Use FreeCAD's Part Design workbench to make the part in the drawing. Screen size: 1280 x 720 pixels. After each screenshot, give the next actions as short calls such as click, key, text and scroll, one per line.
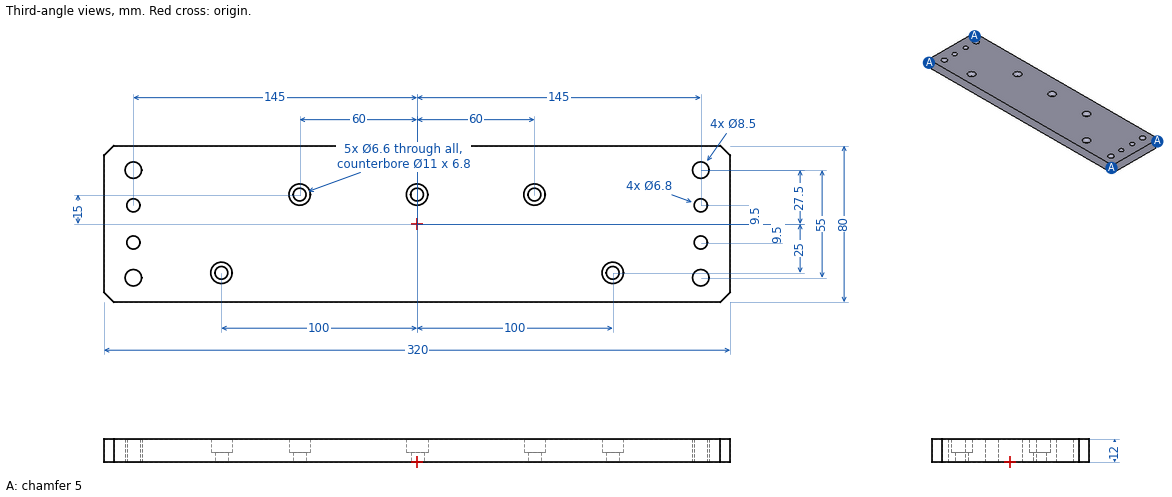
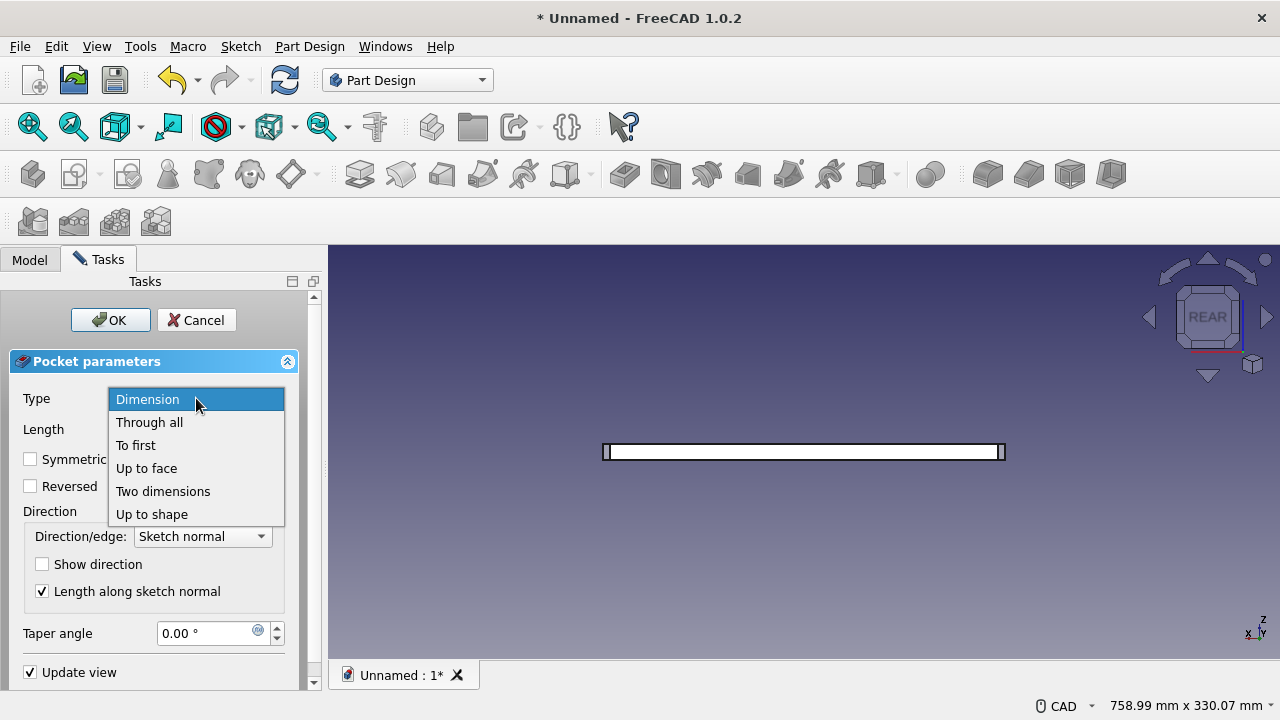
click(194, 422)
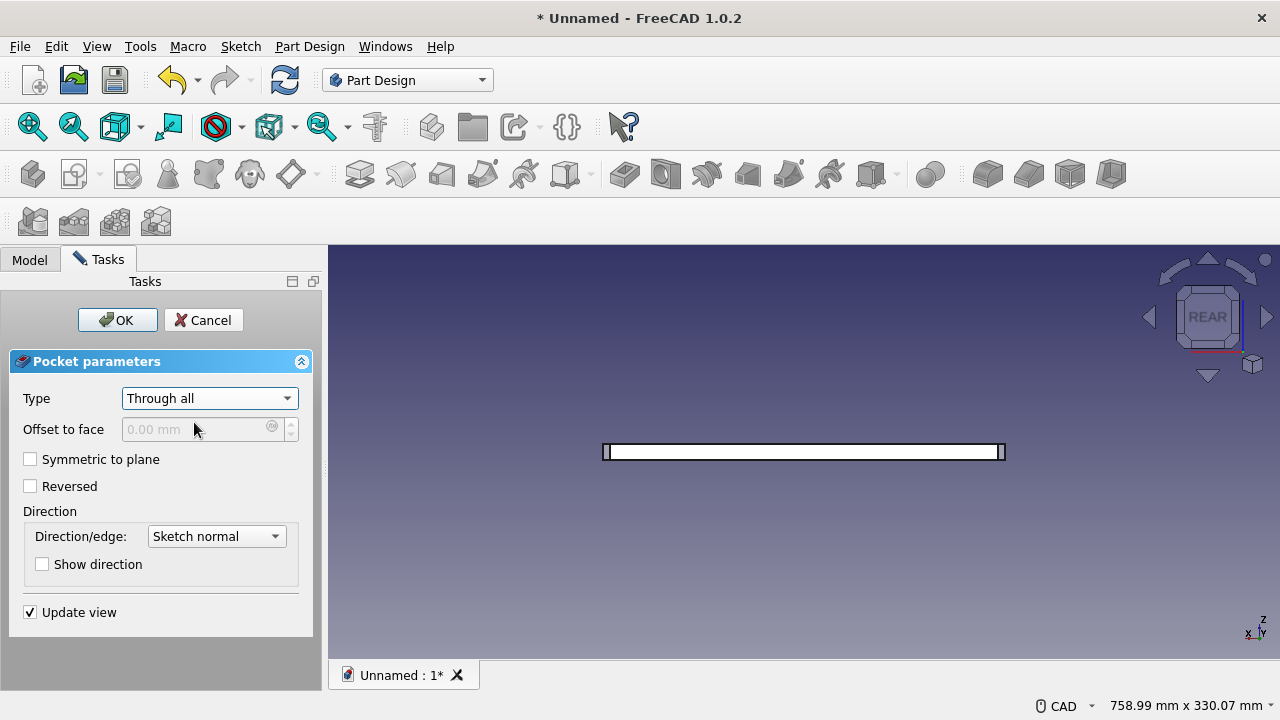
click(31, 486)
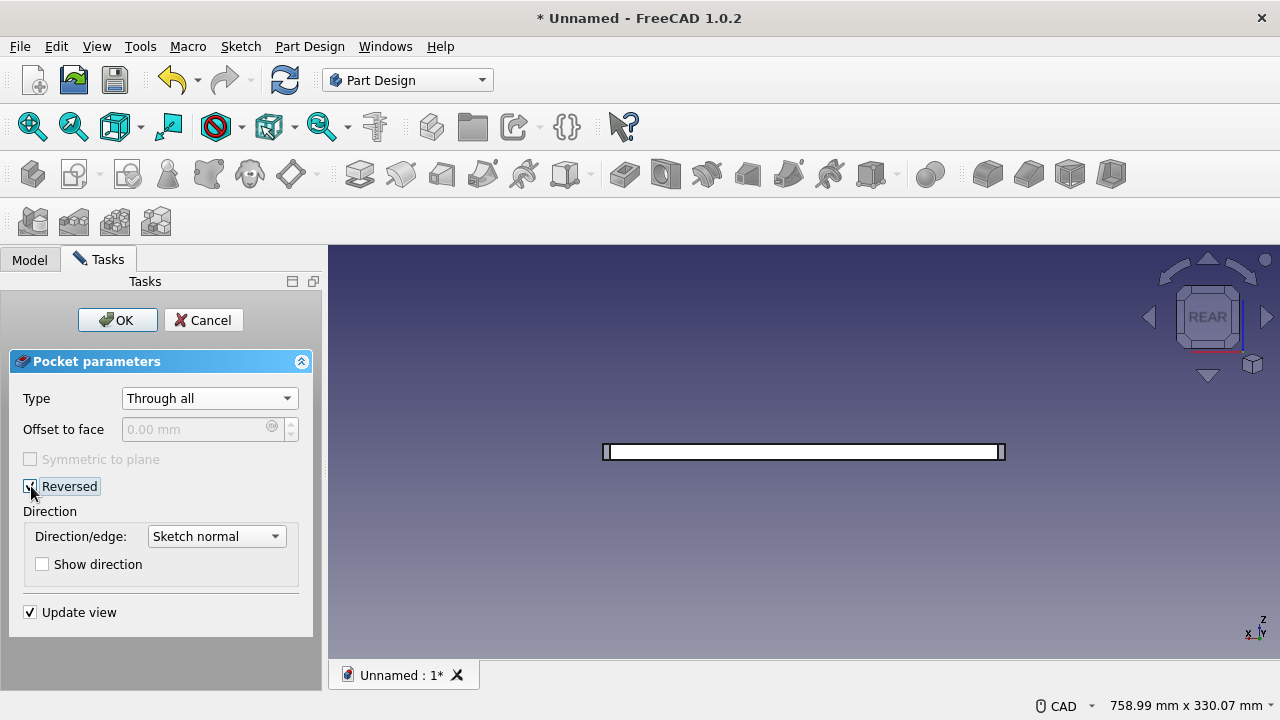
click(118, 320)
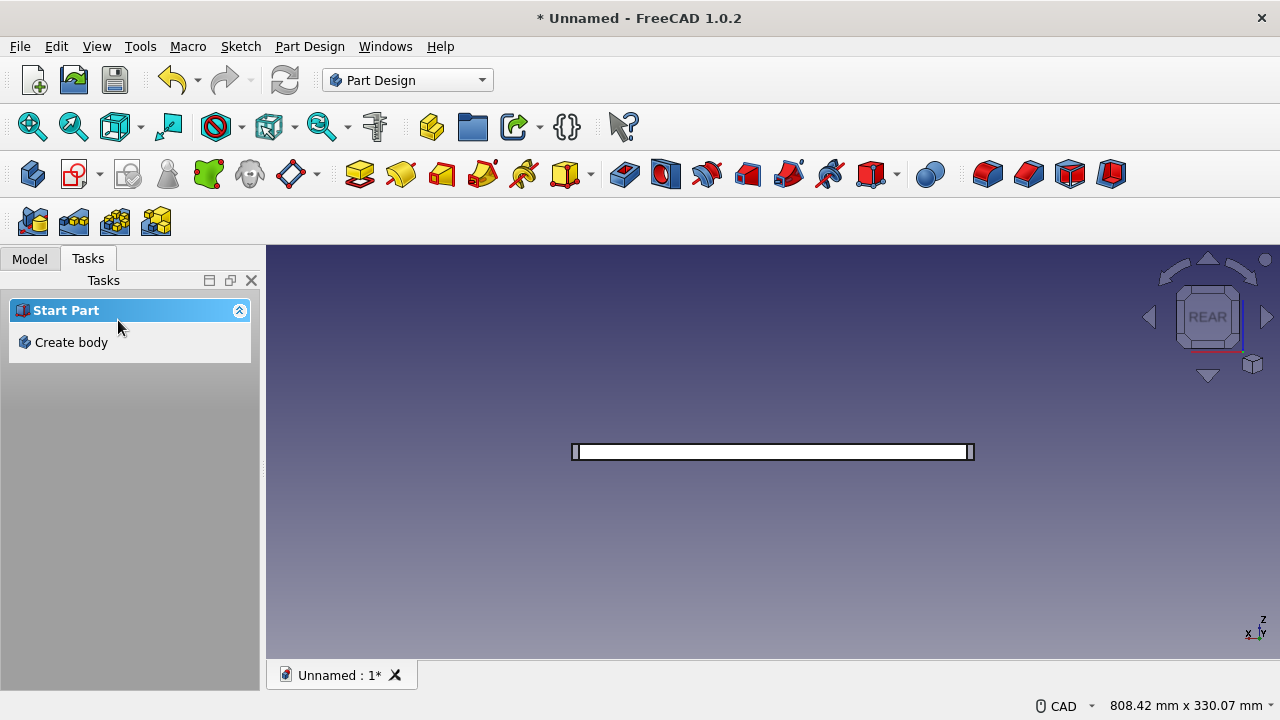
click(33, 128)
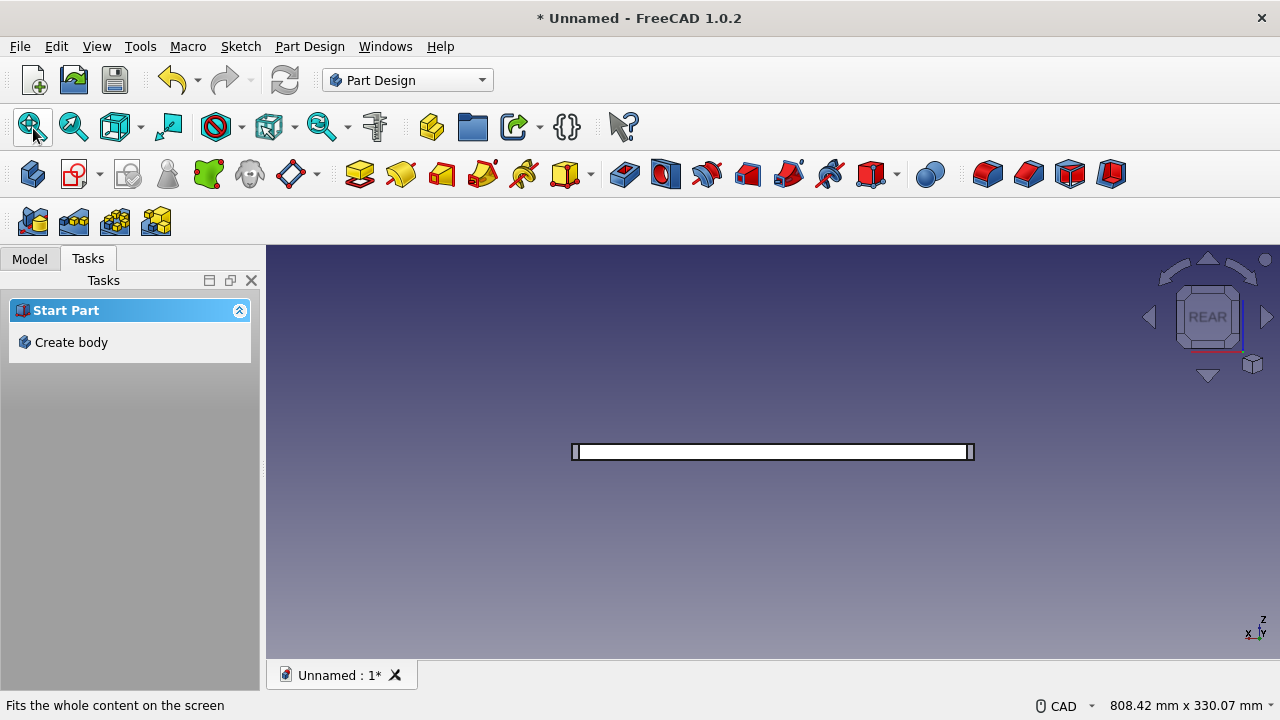
key(5)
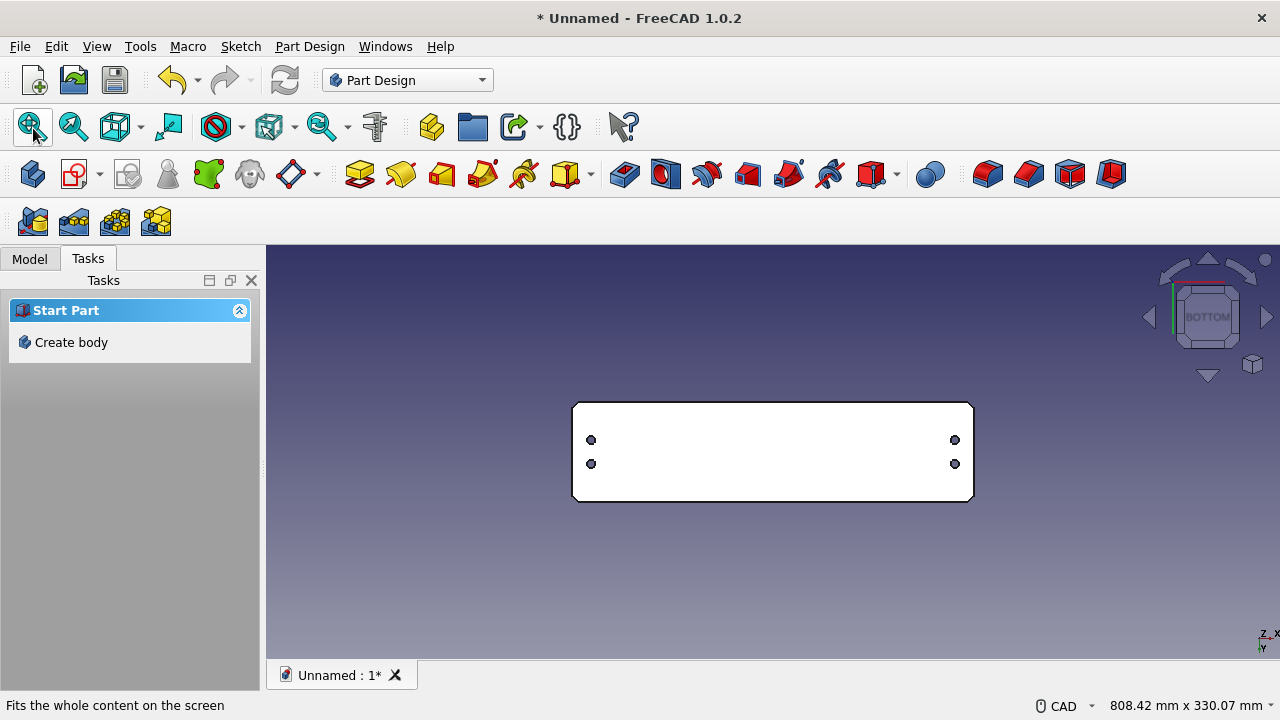
click(33, 128)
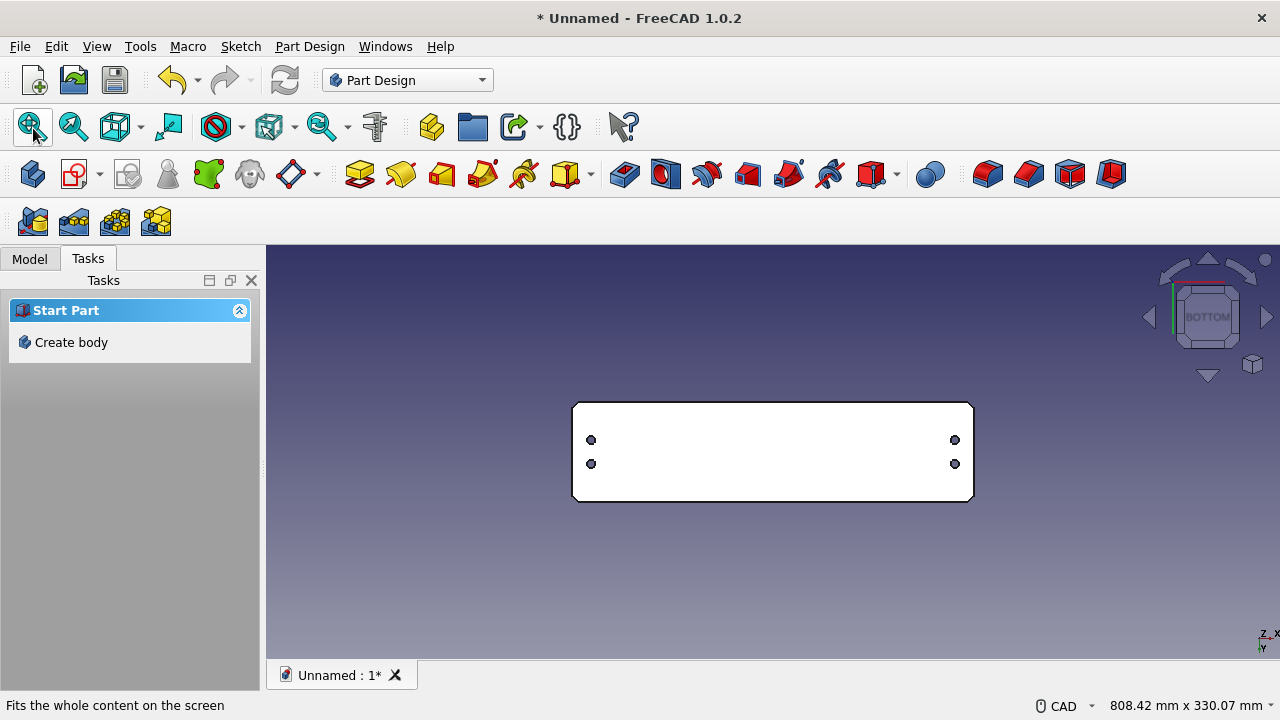
click(888, 451)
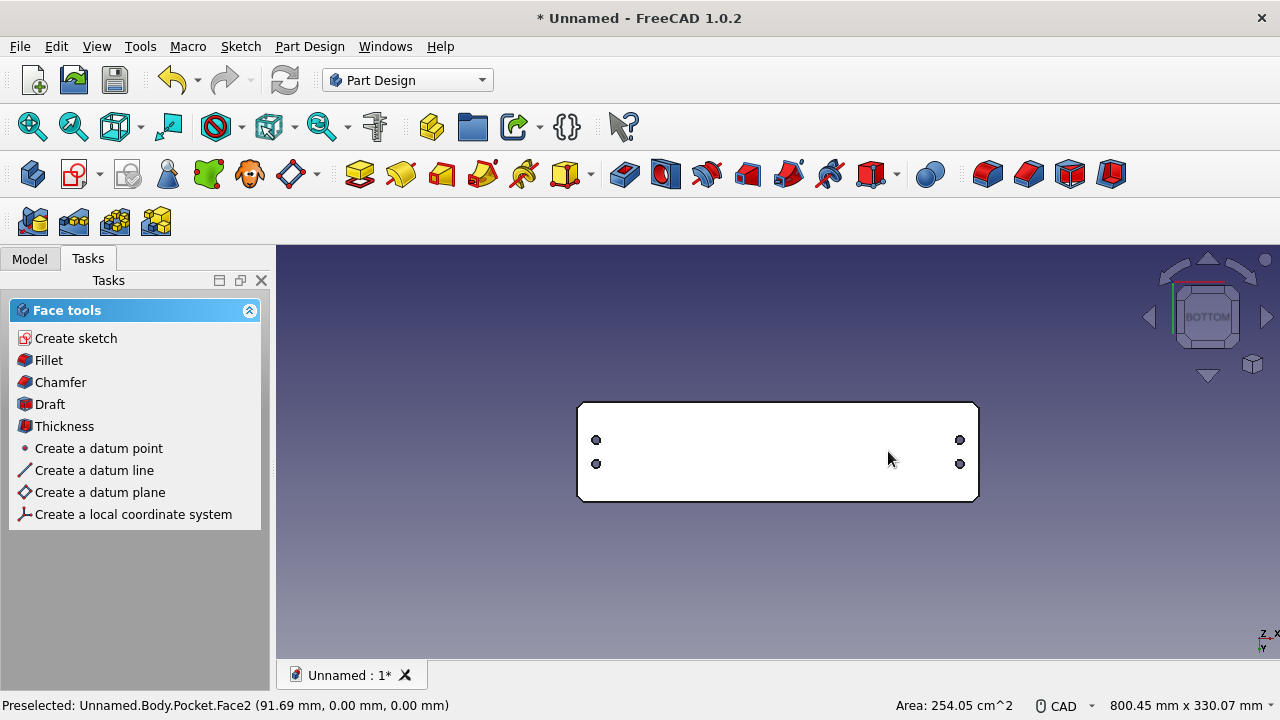
click(74, 174)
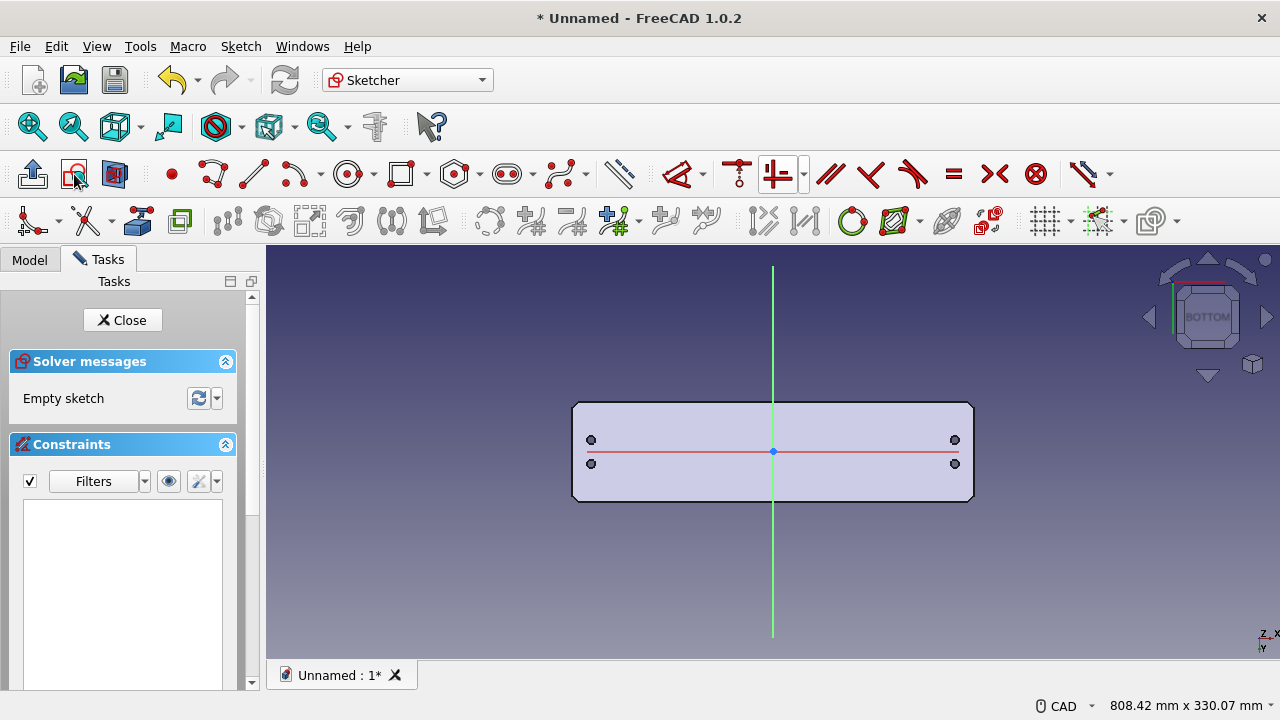
scroll(912, 452, up, 2)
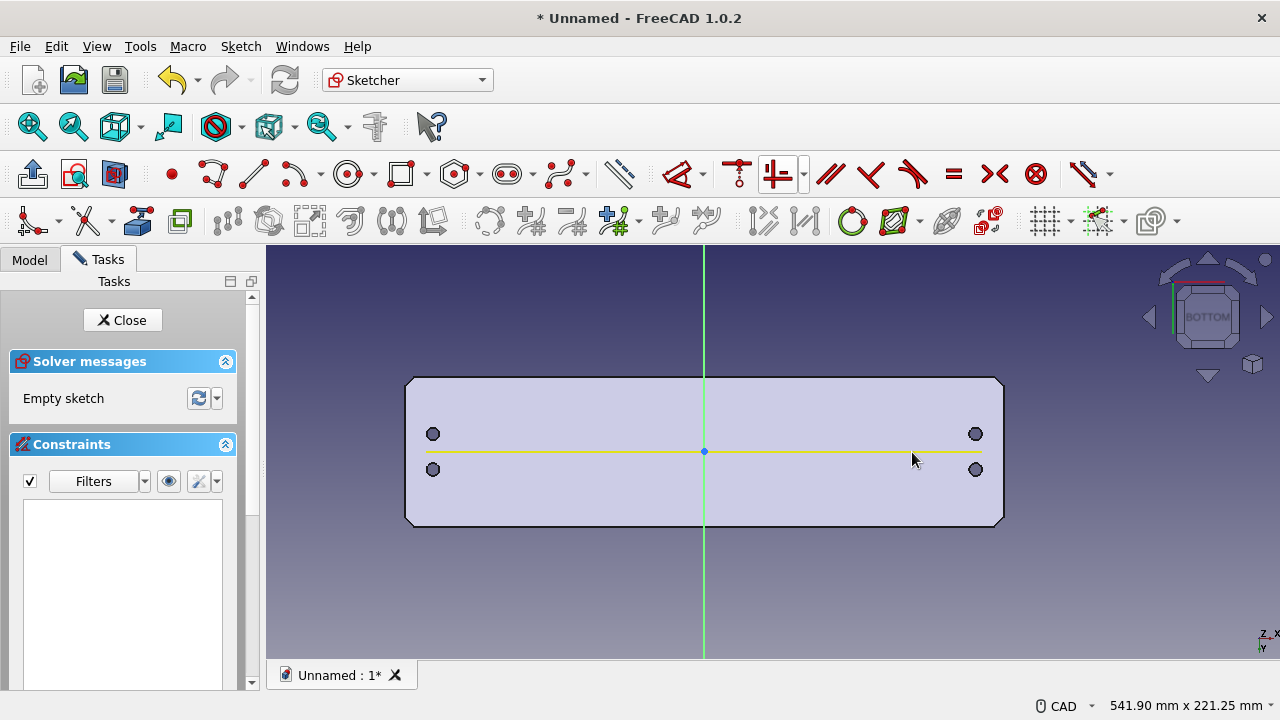
click(348, 174)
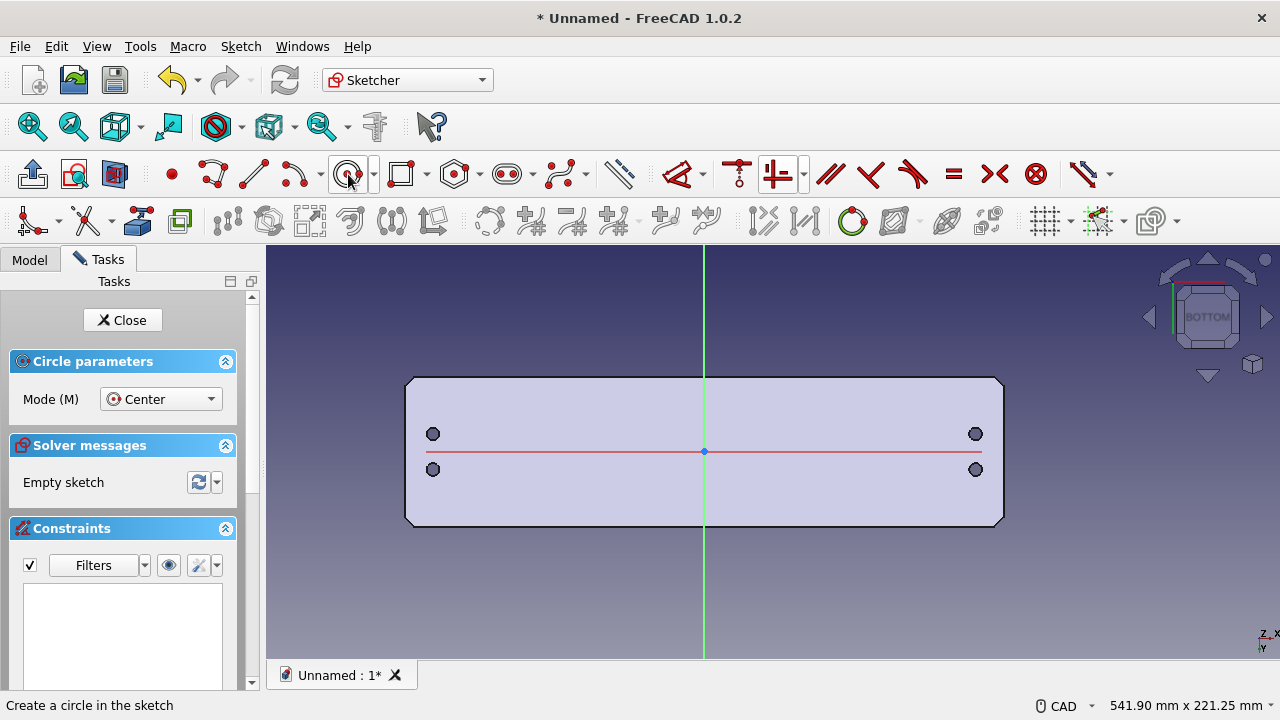
scroll(976, 503, up, 6)